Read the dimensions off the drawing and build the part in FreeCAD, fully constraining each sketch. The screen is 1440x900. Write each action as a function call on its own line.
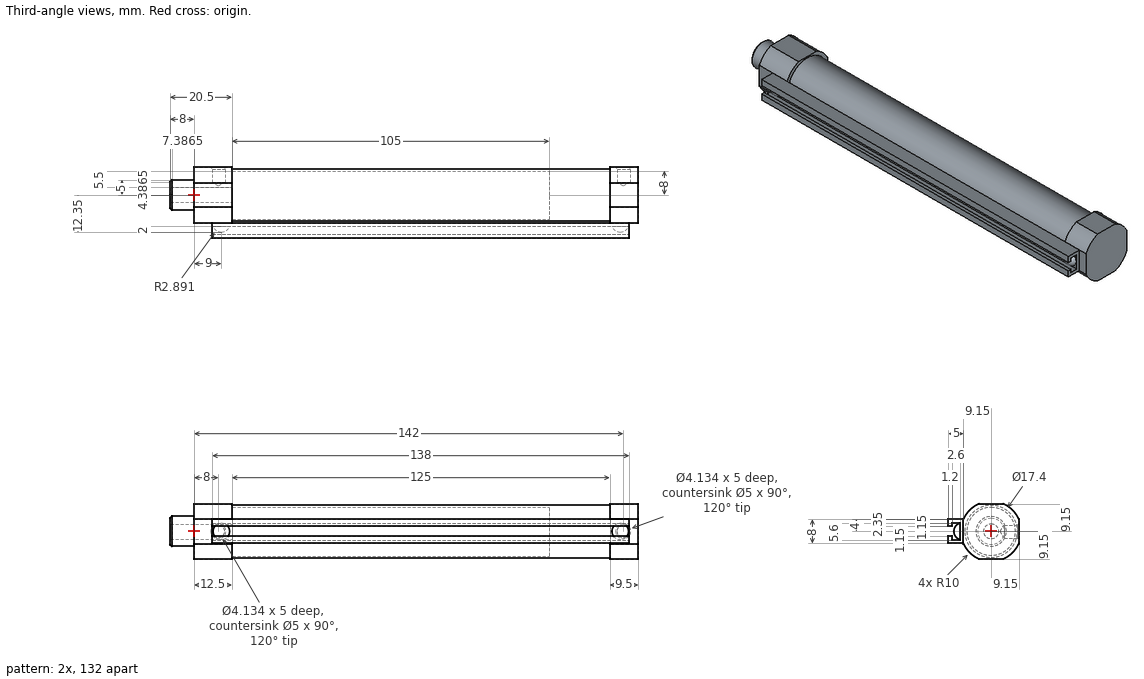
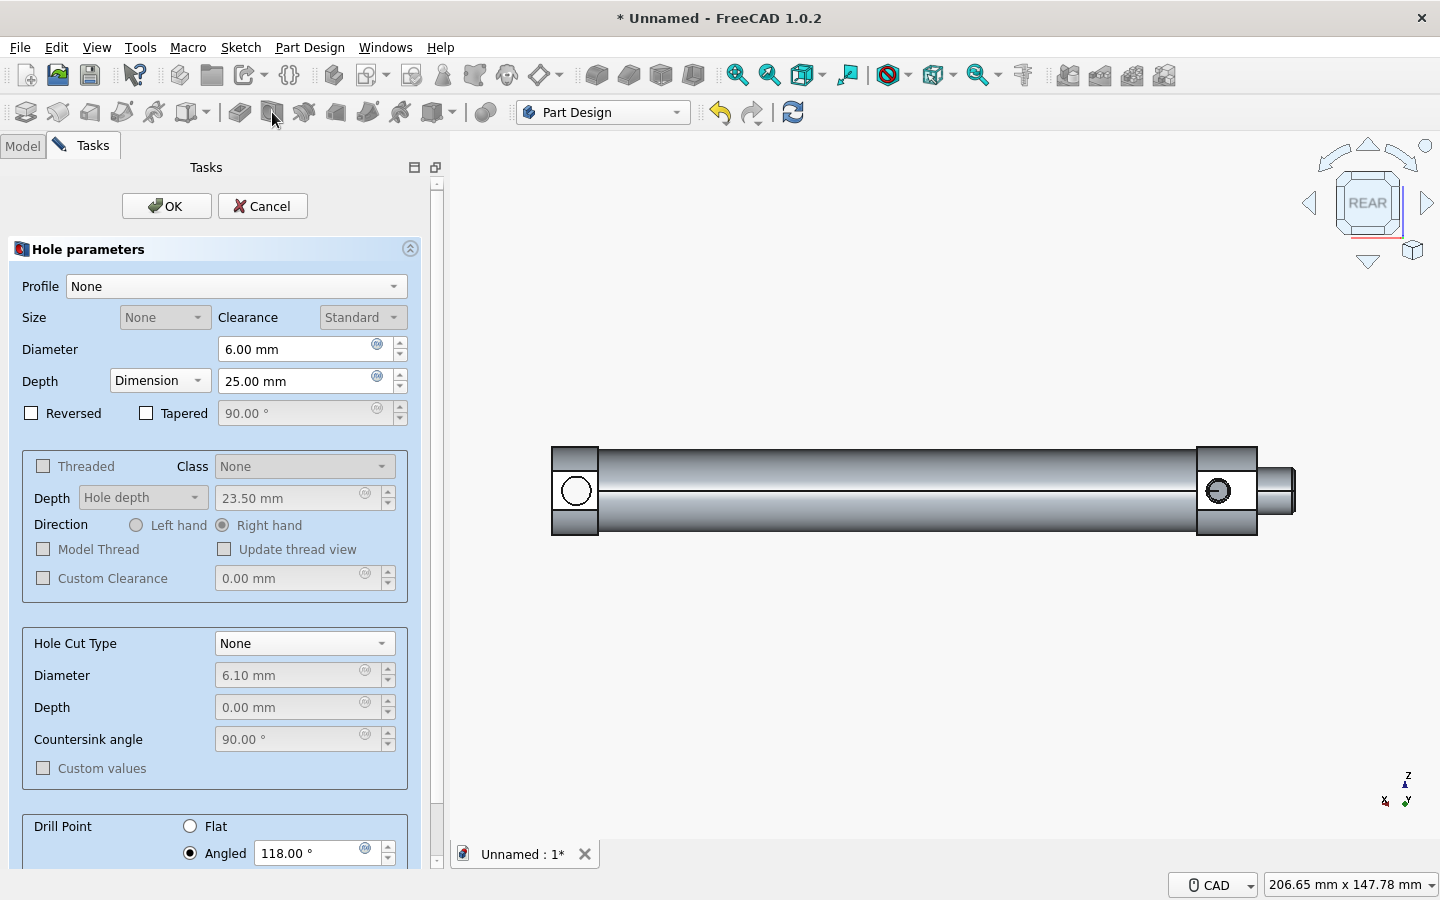
triple_click(305, 349)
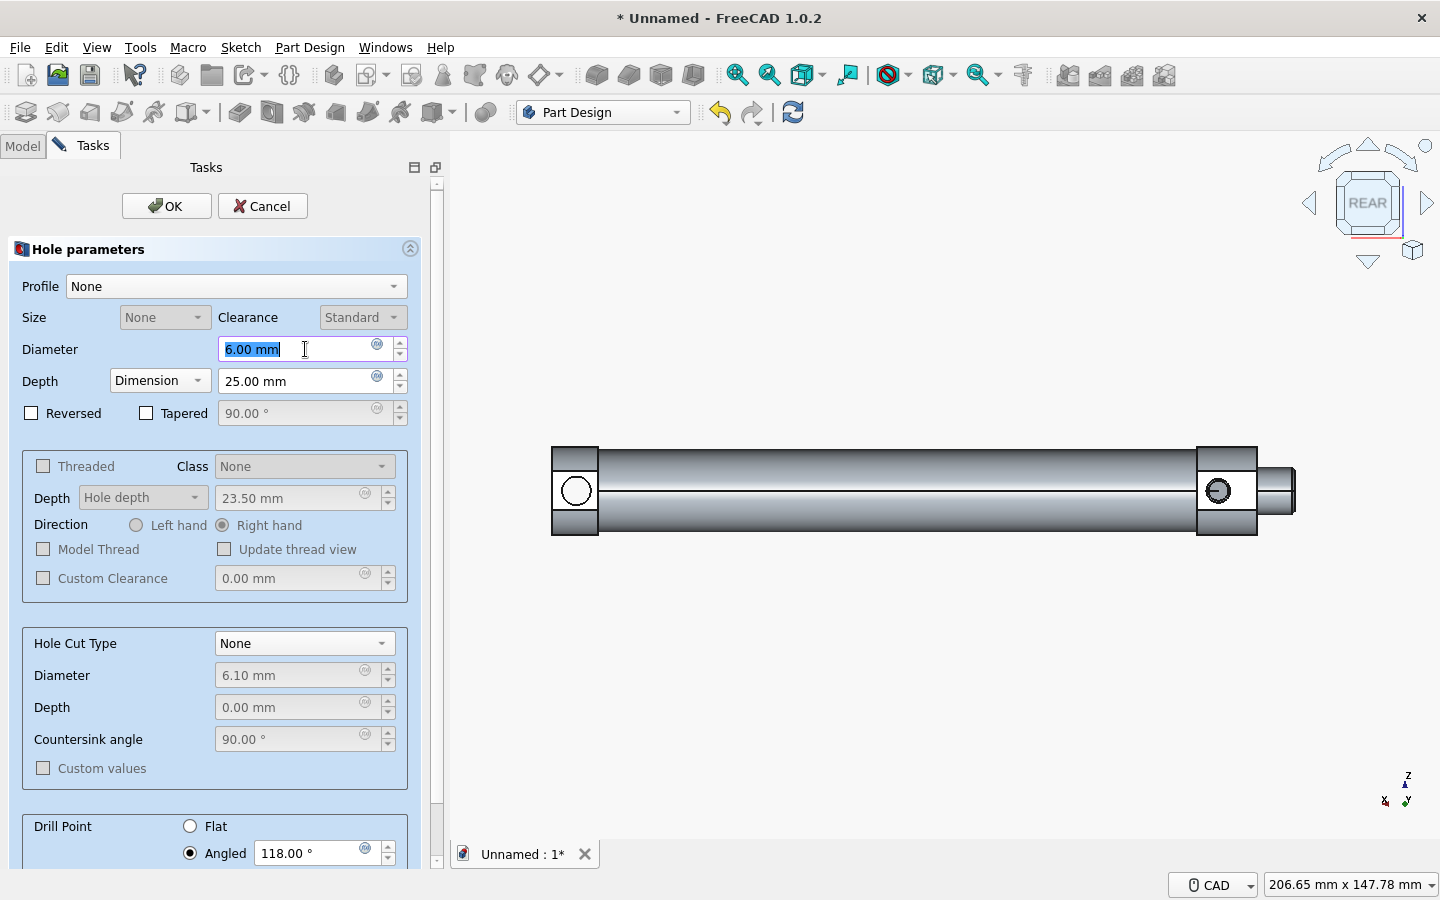
text(4.134)
key(Tab)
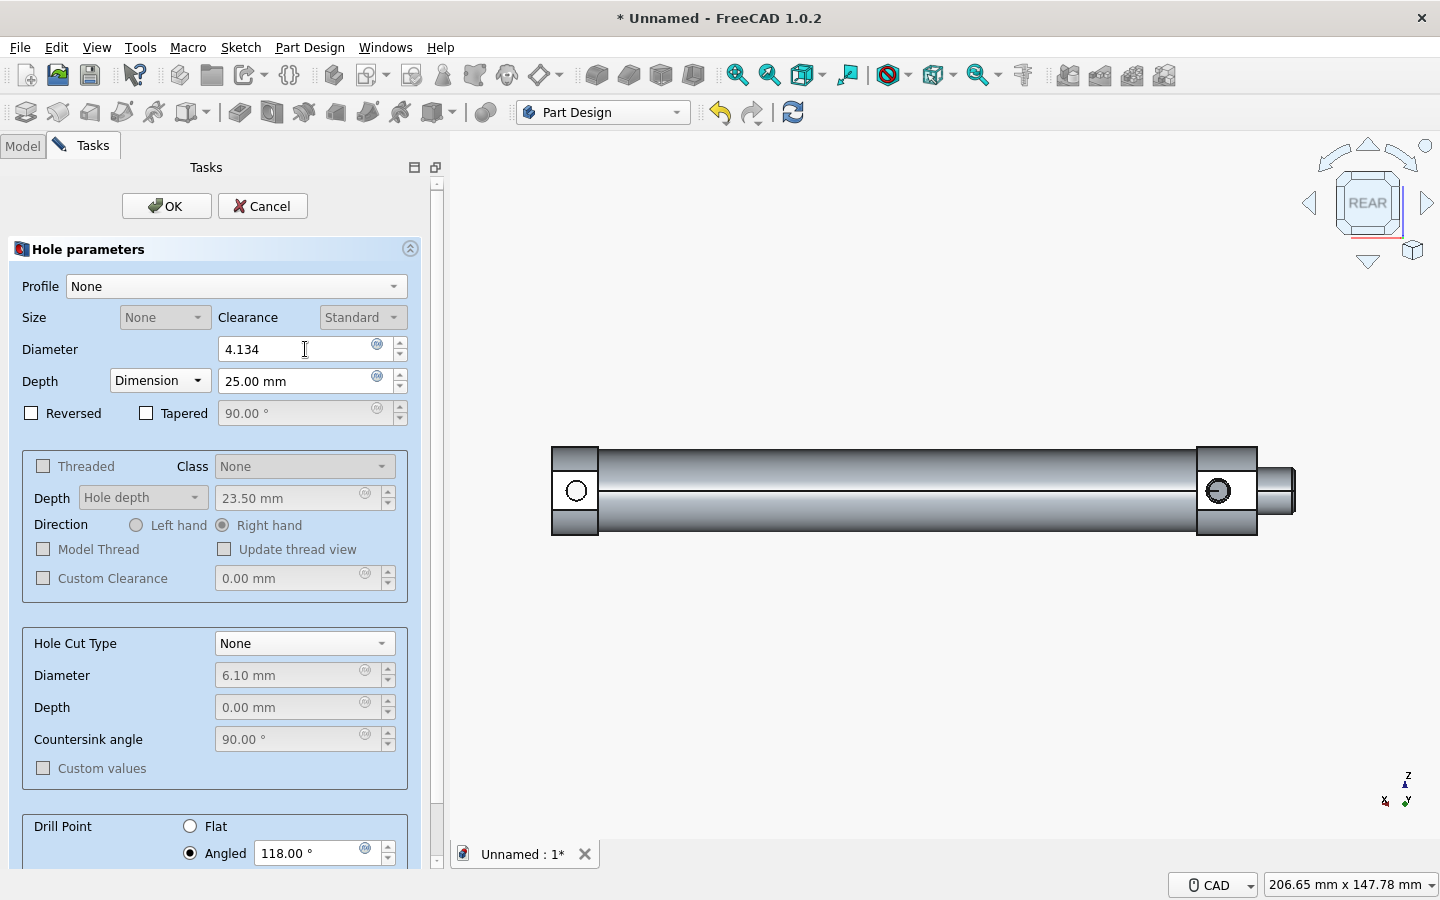
triple_click(305, 381)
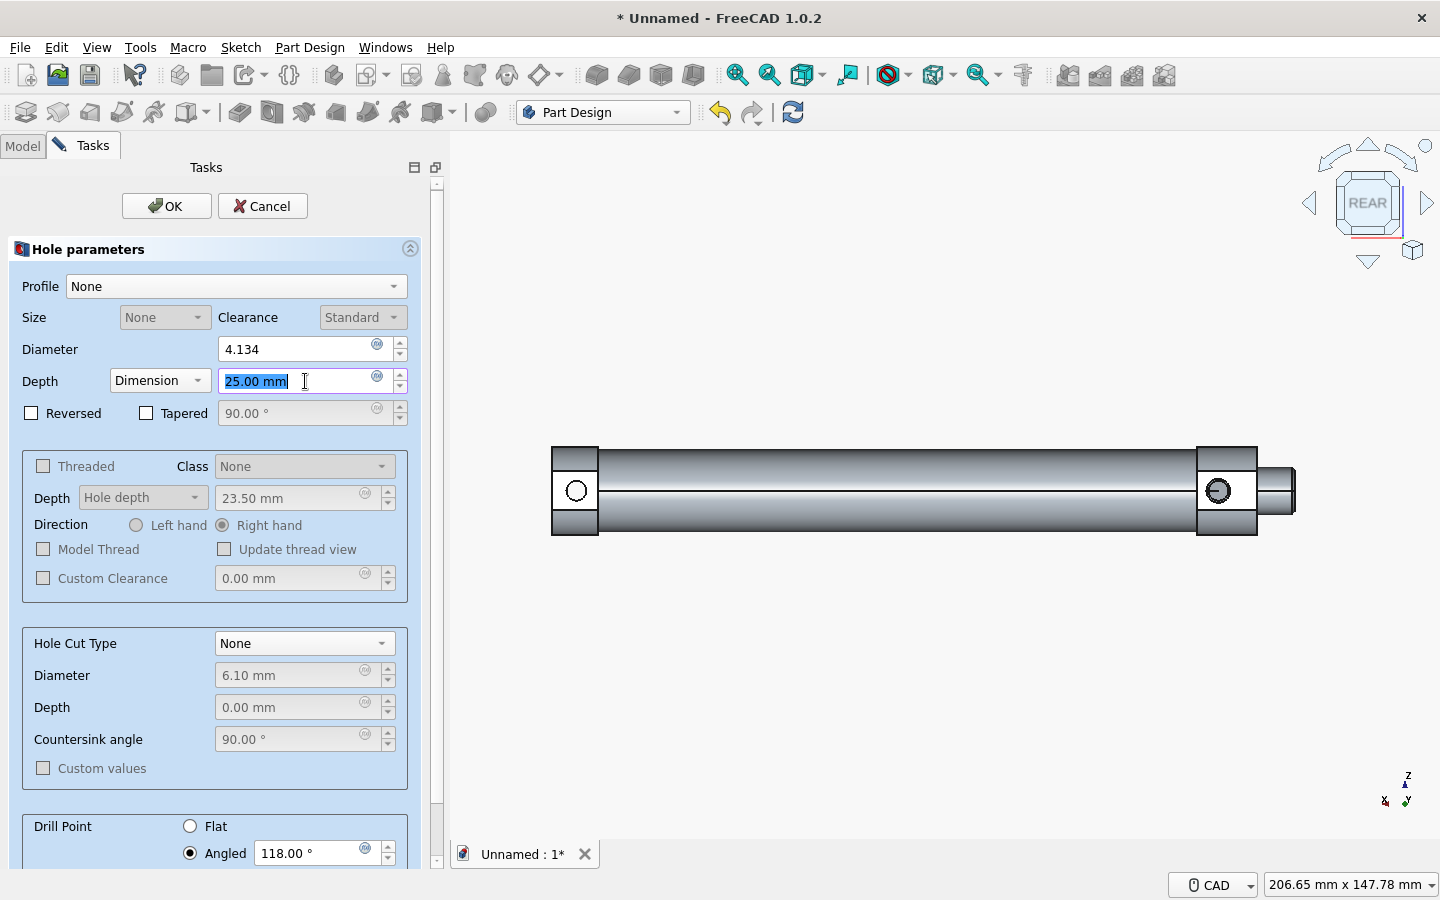
text(5)
key(Tab)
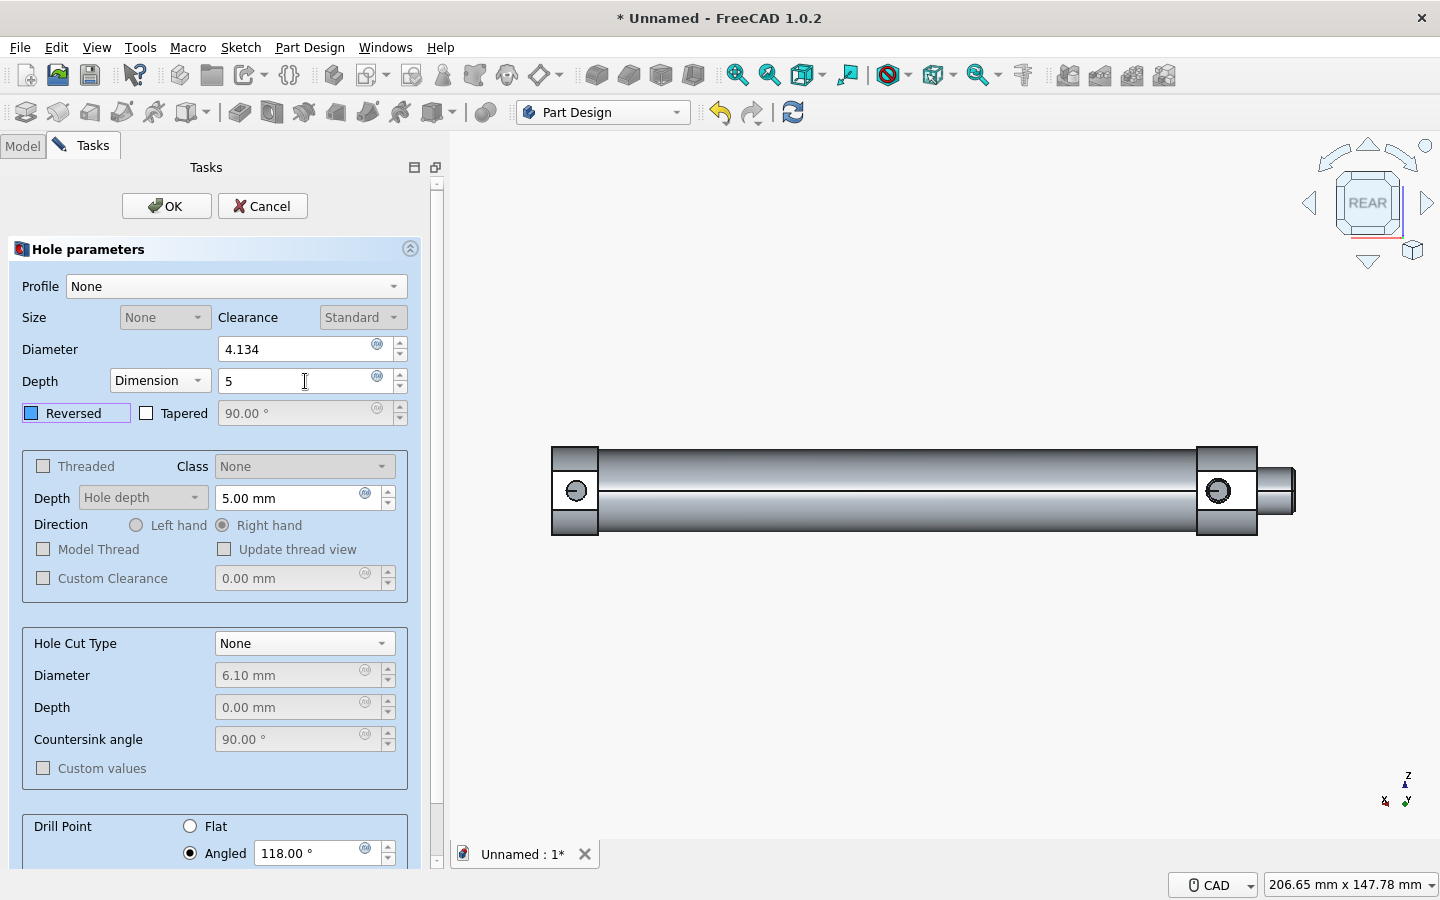
click(306, 644)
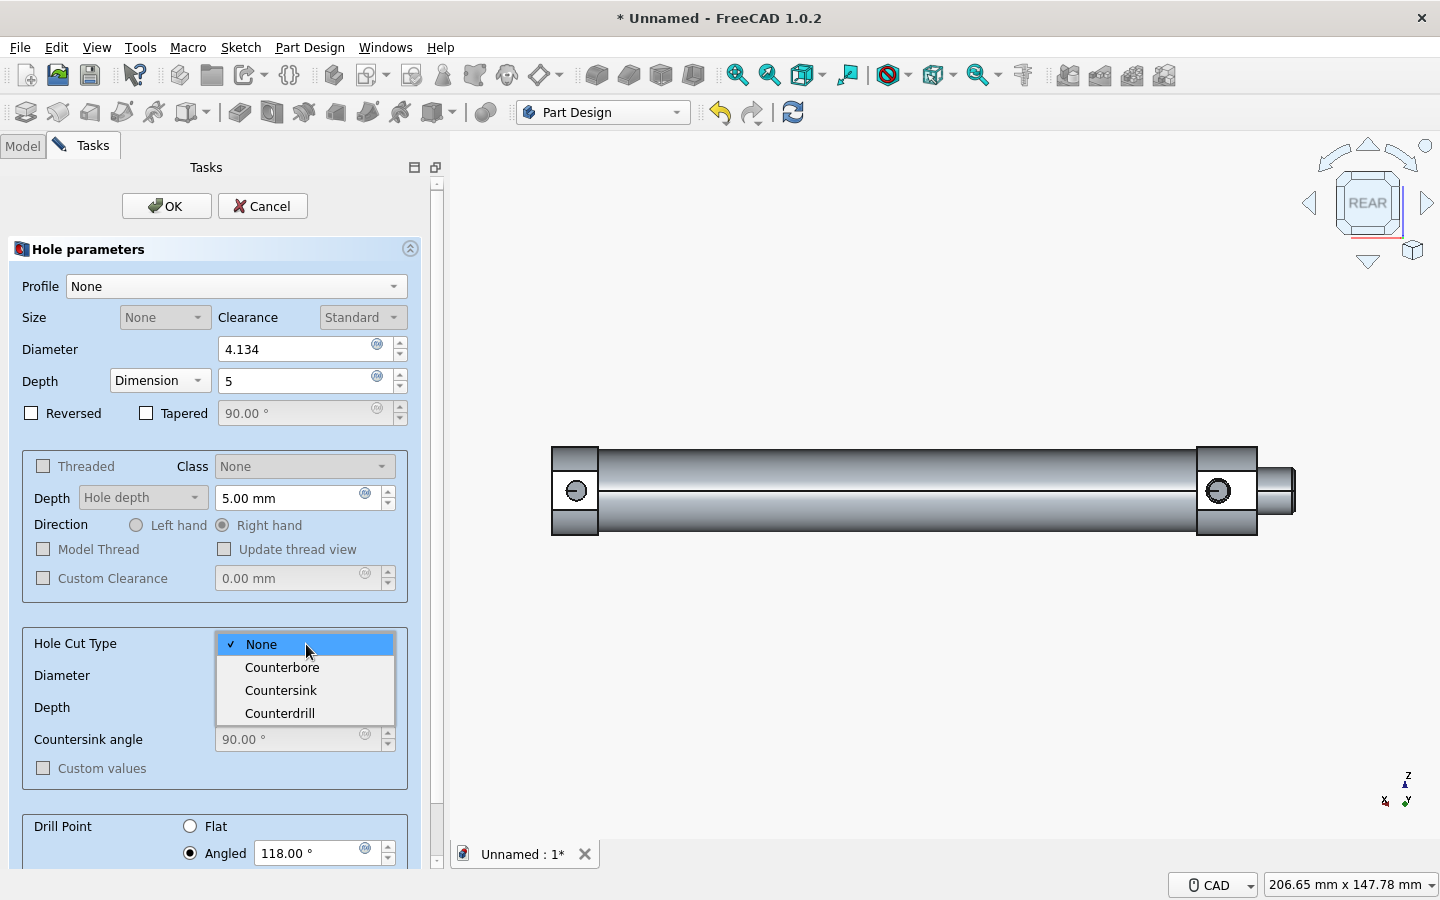
click(304, 690)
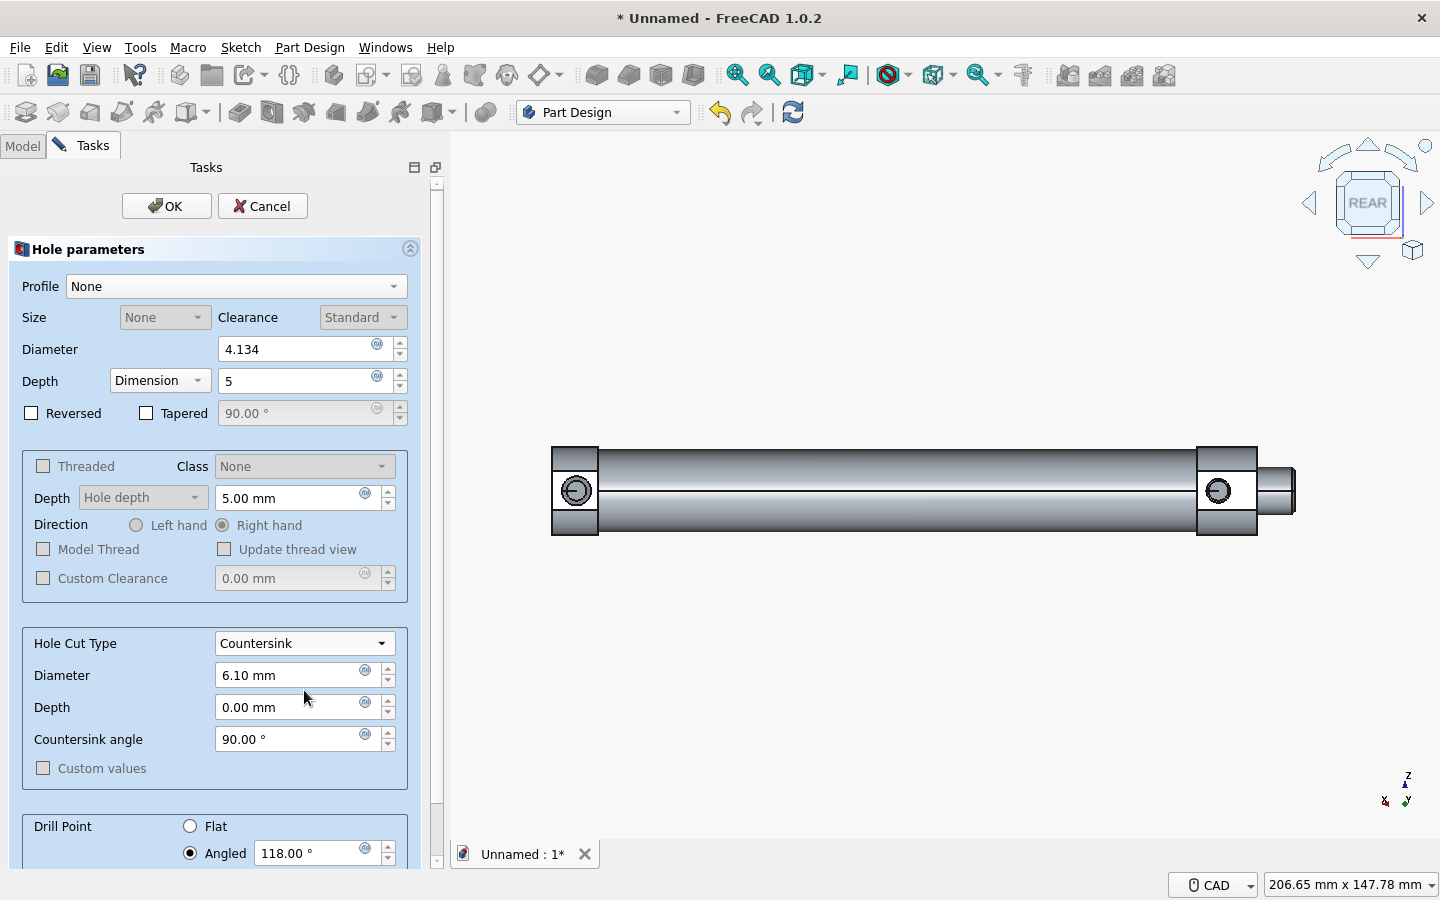
triple_click(298, 675)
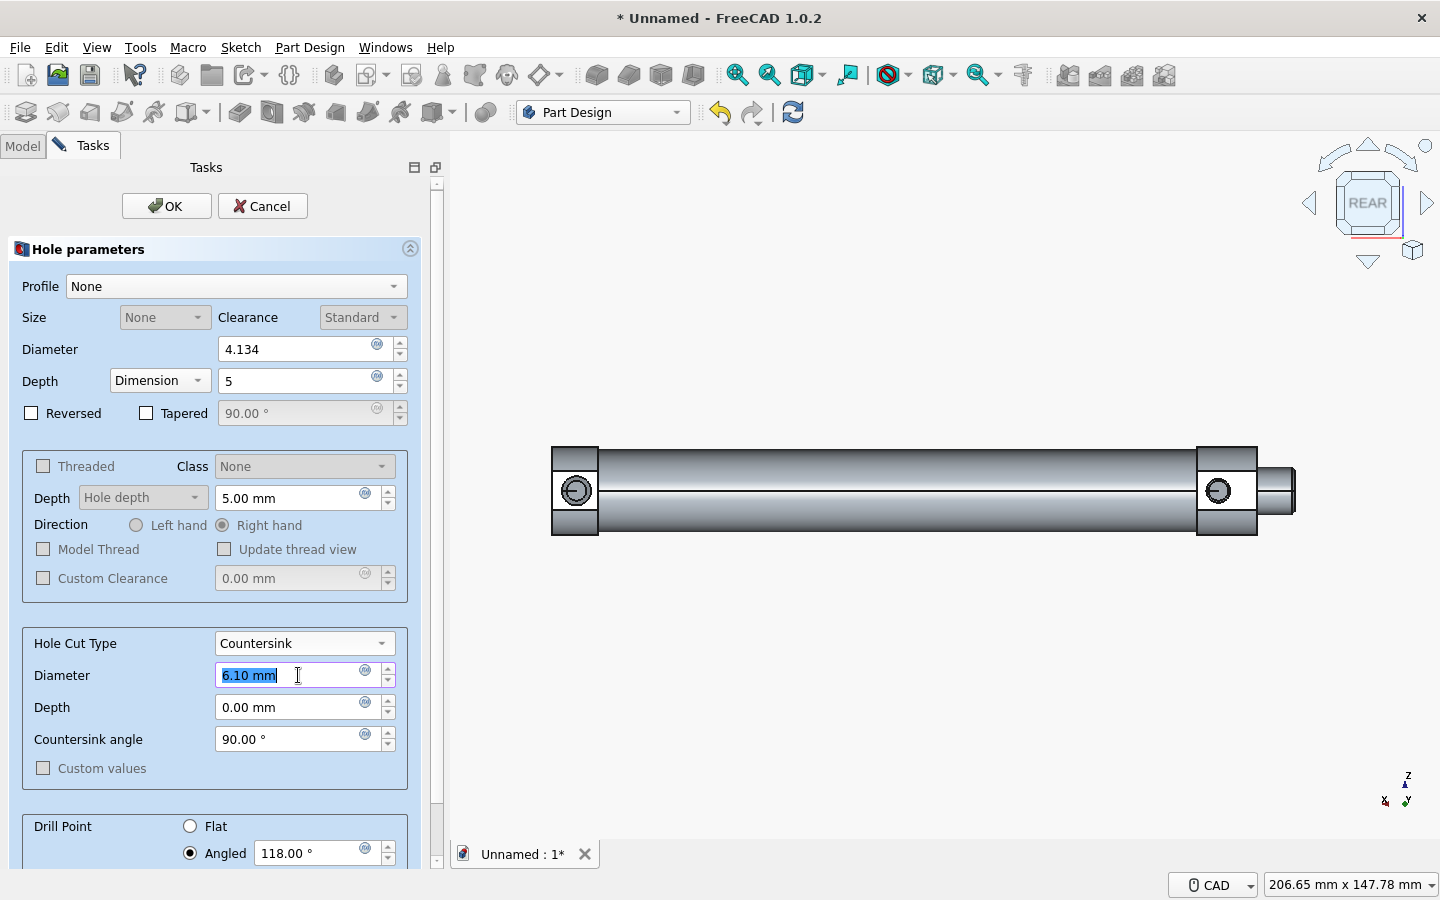
text(5)
key(Tab)